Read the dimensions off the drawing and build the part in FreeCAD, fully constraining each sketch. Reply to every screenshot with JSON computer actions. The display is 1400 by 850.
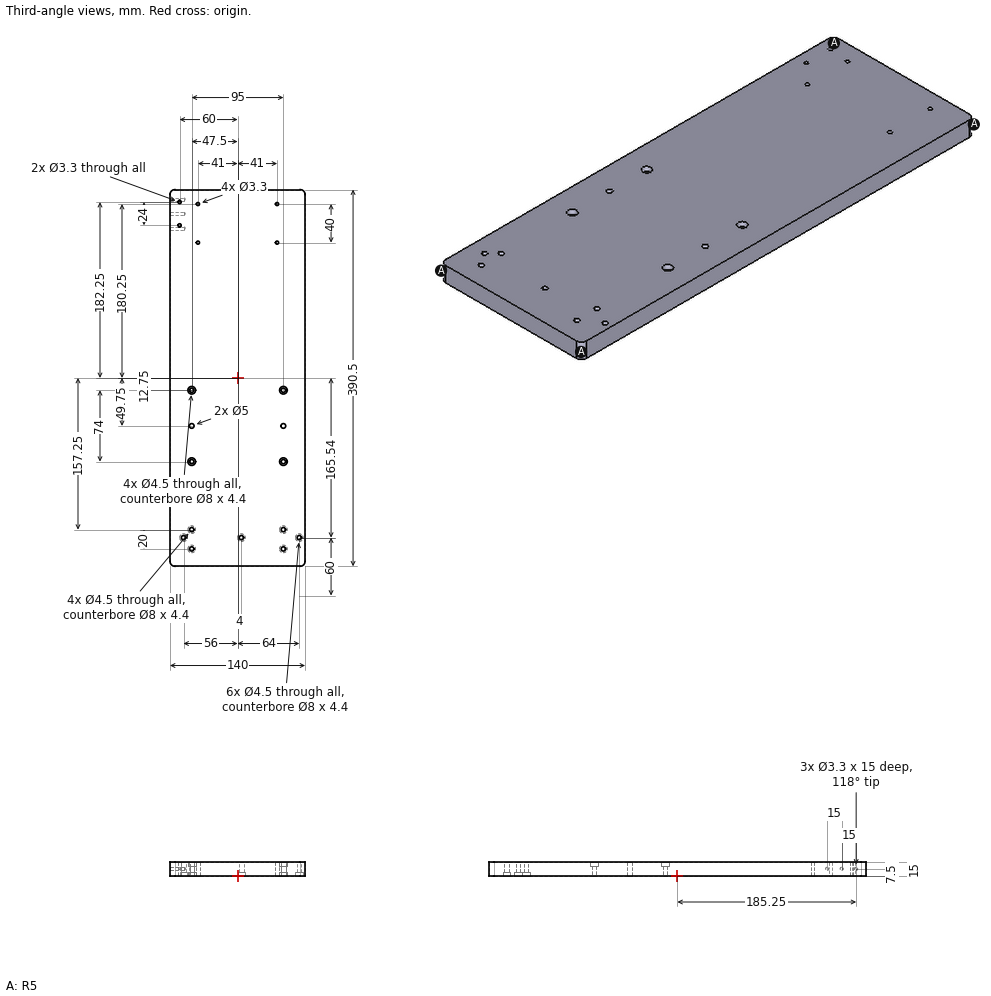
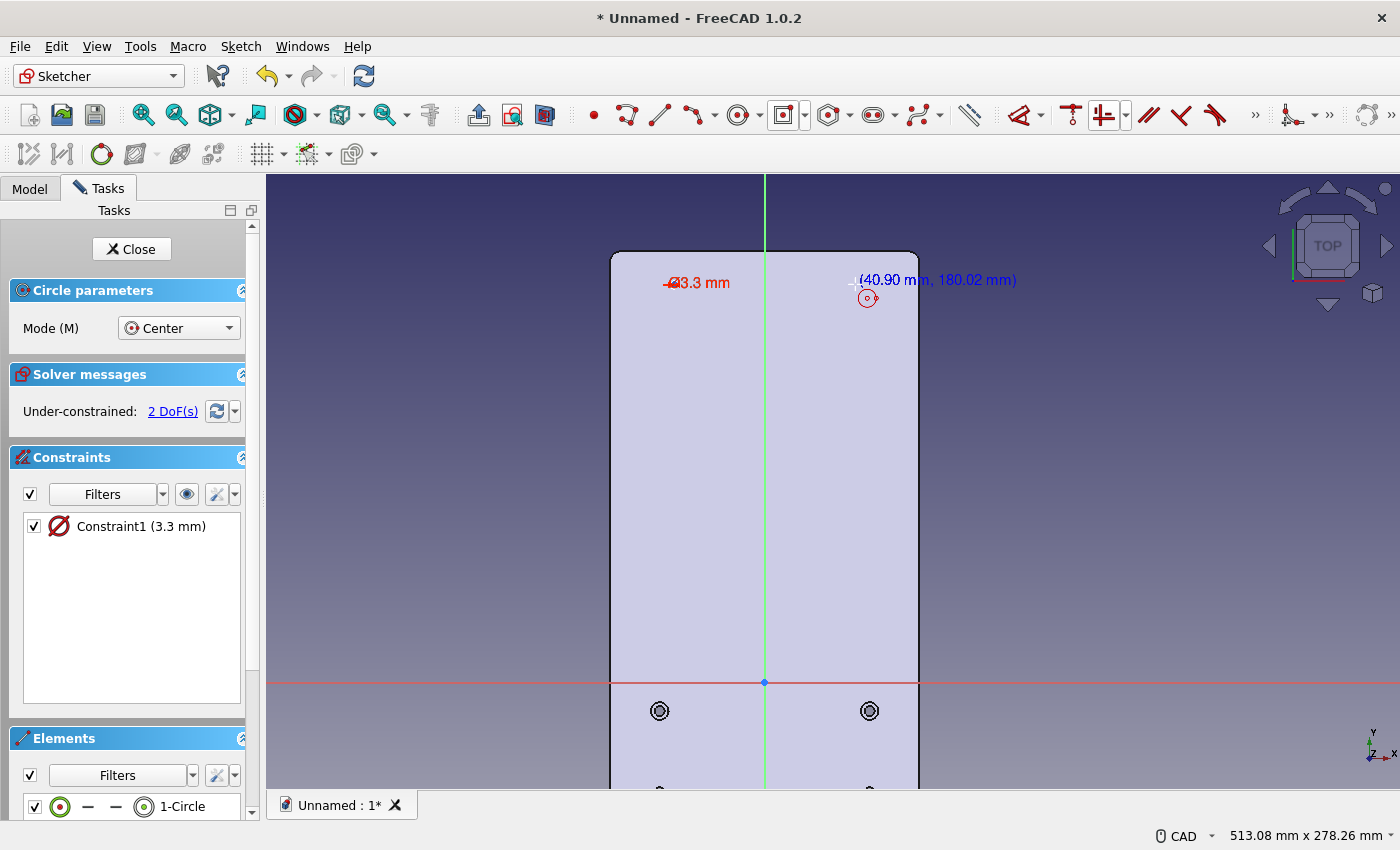
{"action": "left_click", "coordinate": [855, 284]}
{"action": "mouse_move", "coordinate": [858, 282]}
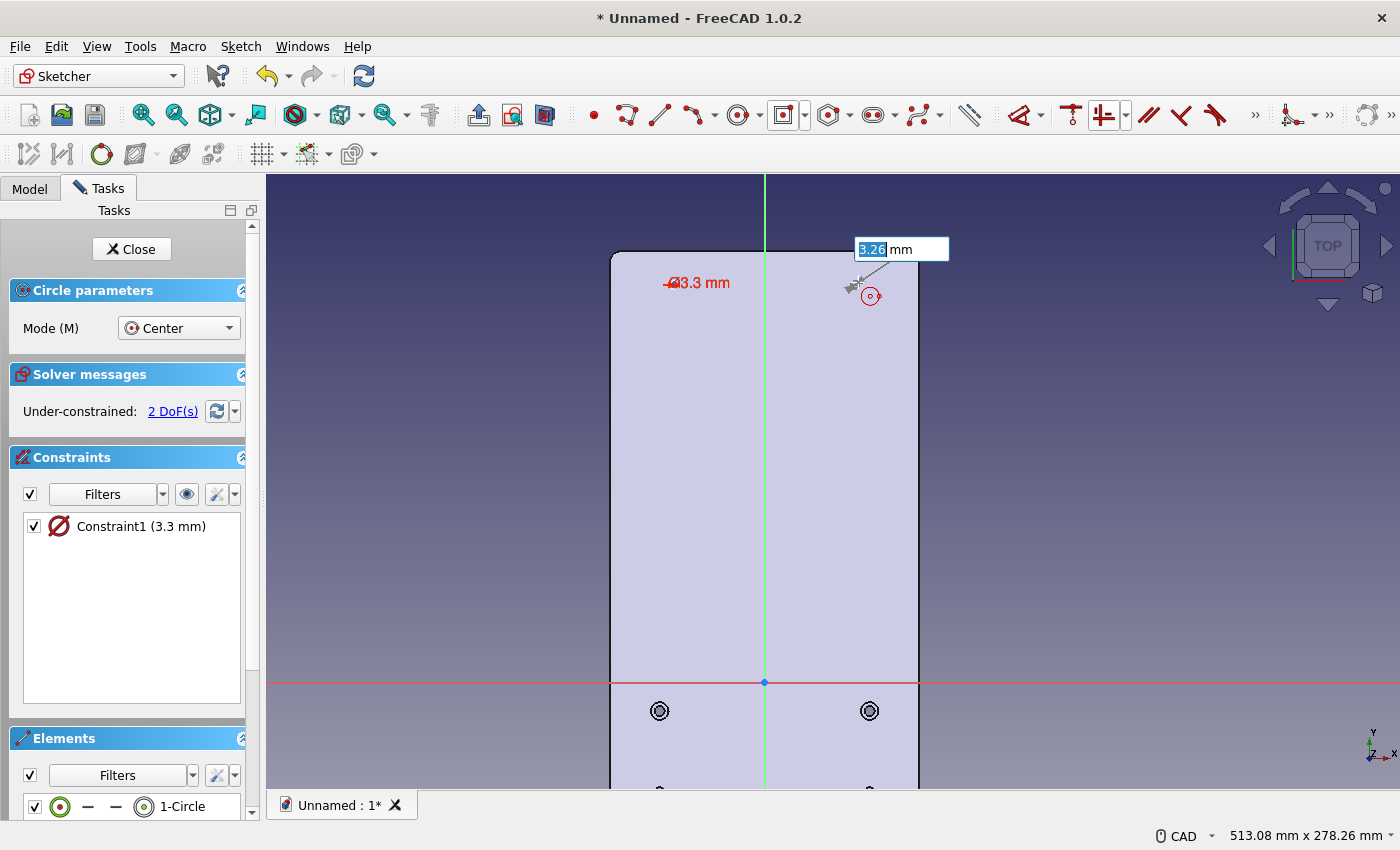
{"action": "type", "text": "3.3"}
{"action": "key", "text": "Return"}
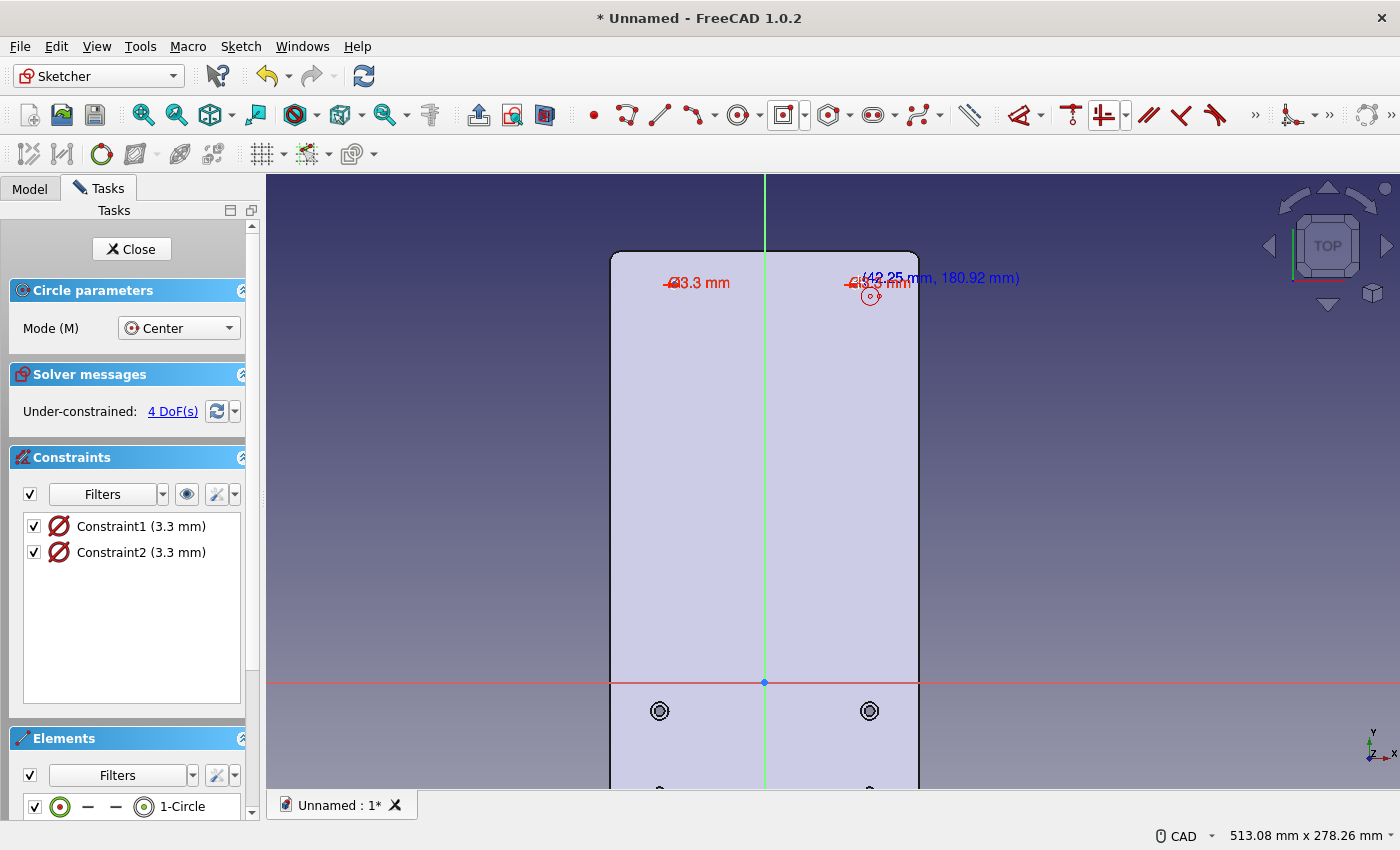
{"action": "scroll", "coordinate": [855, 373], "scroll_direction": "up", "scroll_amount": 10}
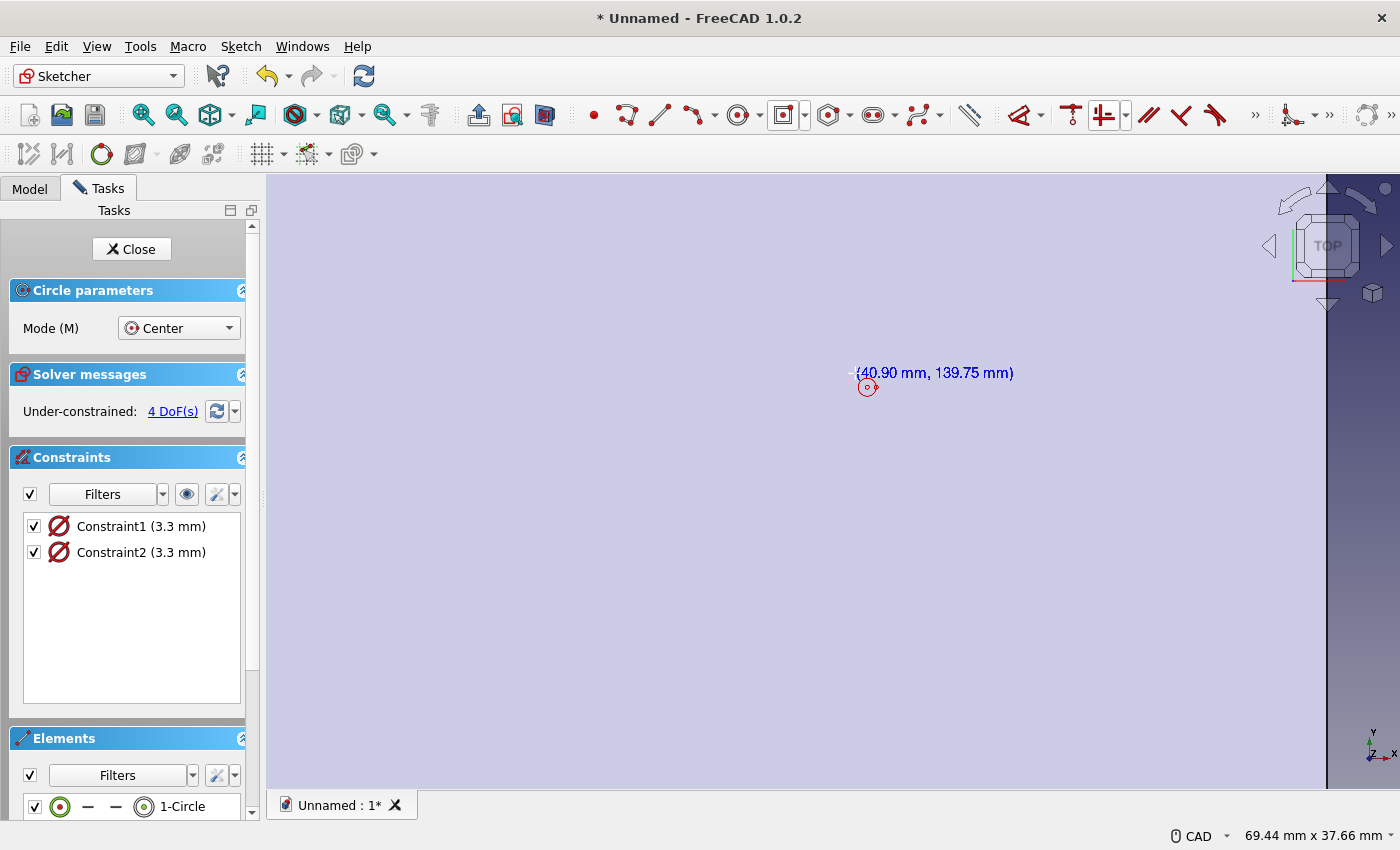
{"action": "scroll", "coordinate": [855, 373], "scroll_direction": "down", "scroll_amount": 10}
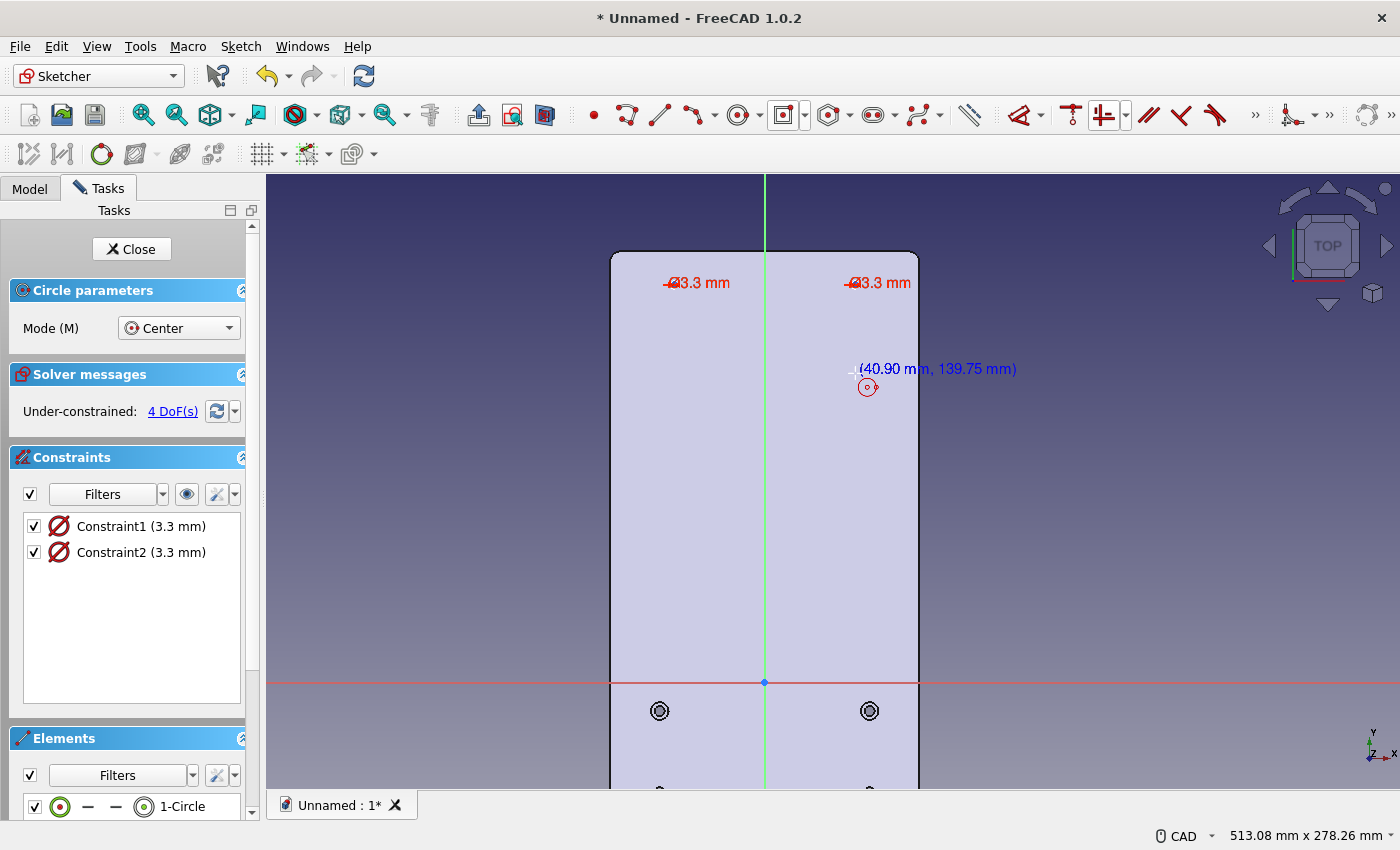
{"action": "left_click", "coordinate": [855, 373]}
{"action": "mouse_move", "coordinate": [858, 370]}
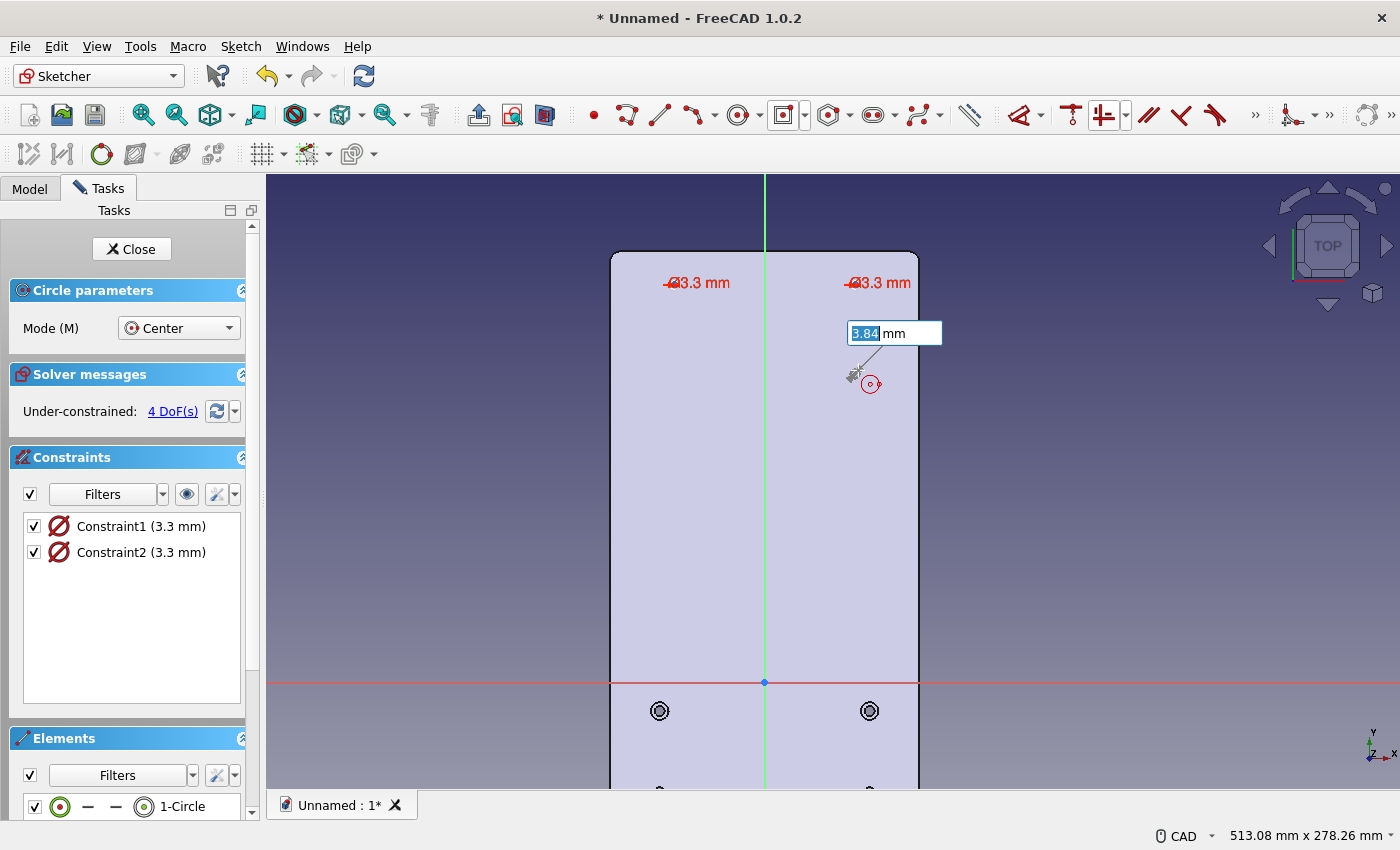
{"action": "type", "text": "3.3"}
{"action": "key", "text": "Return"}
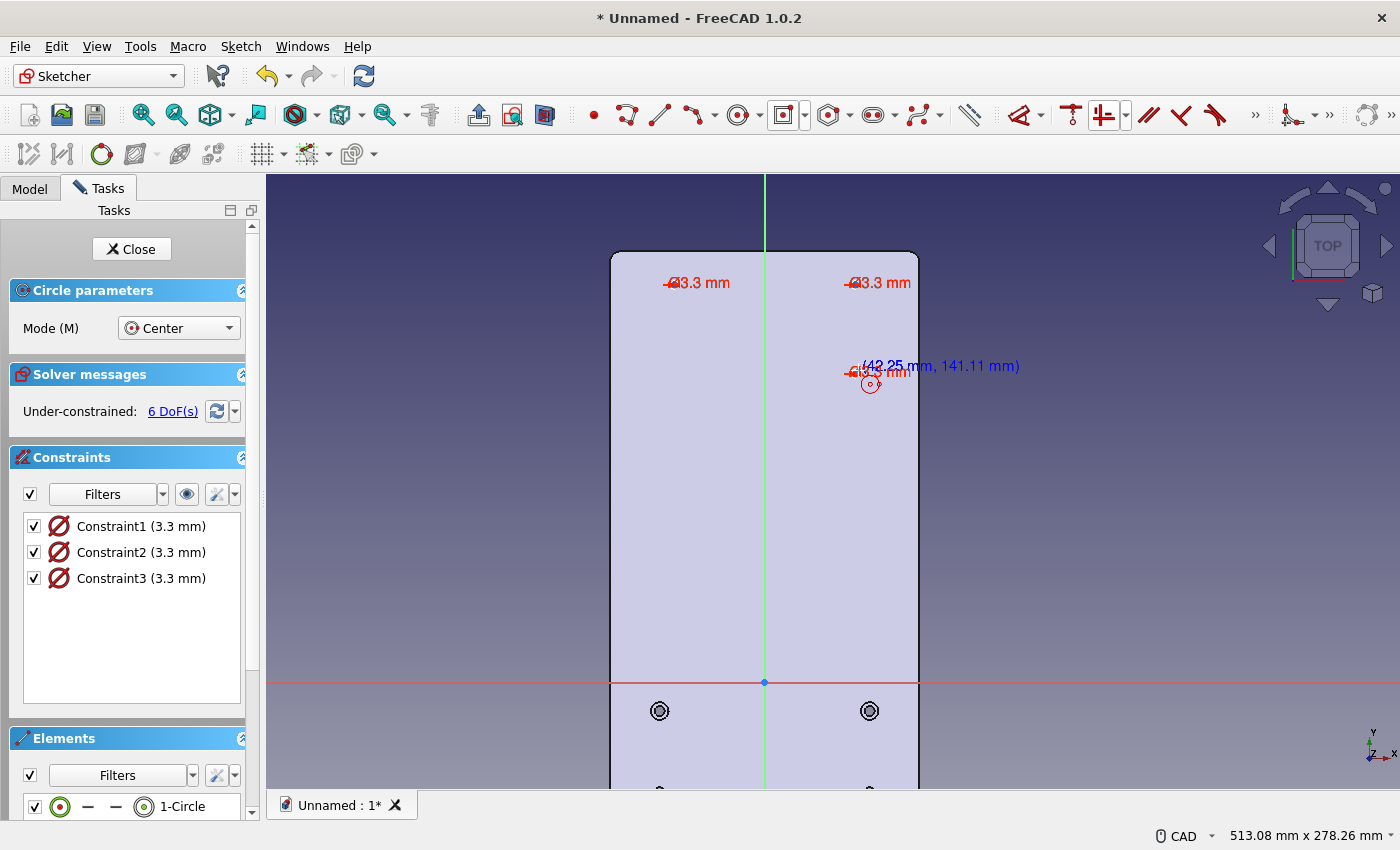
{"action": "scroll", "coordinate": [674, 373], "scroll_direction": "up", "scroll_amount": 10}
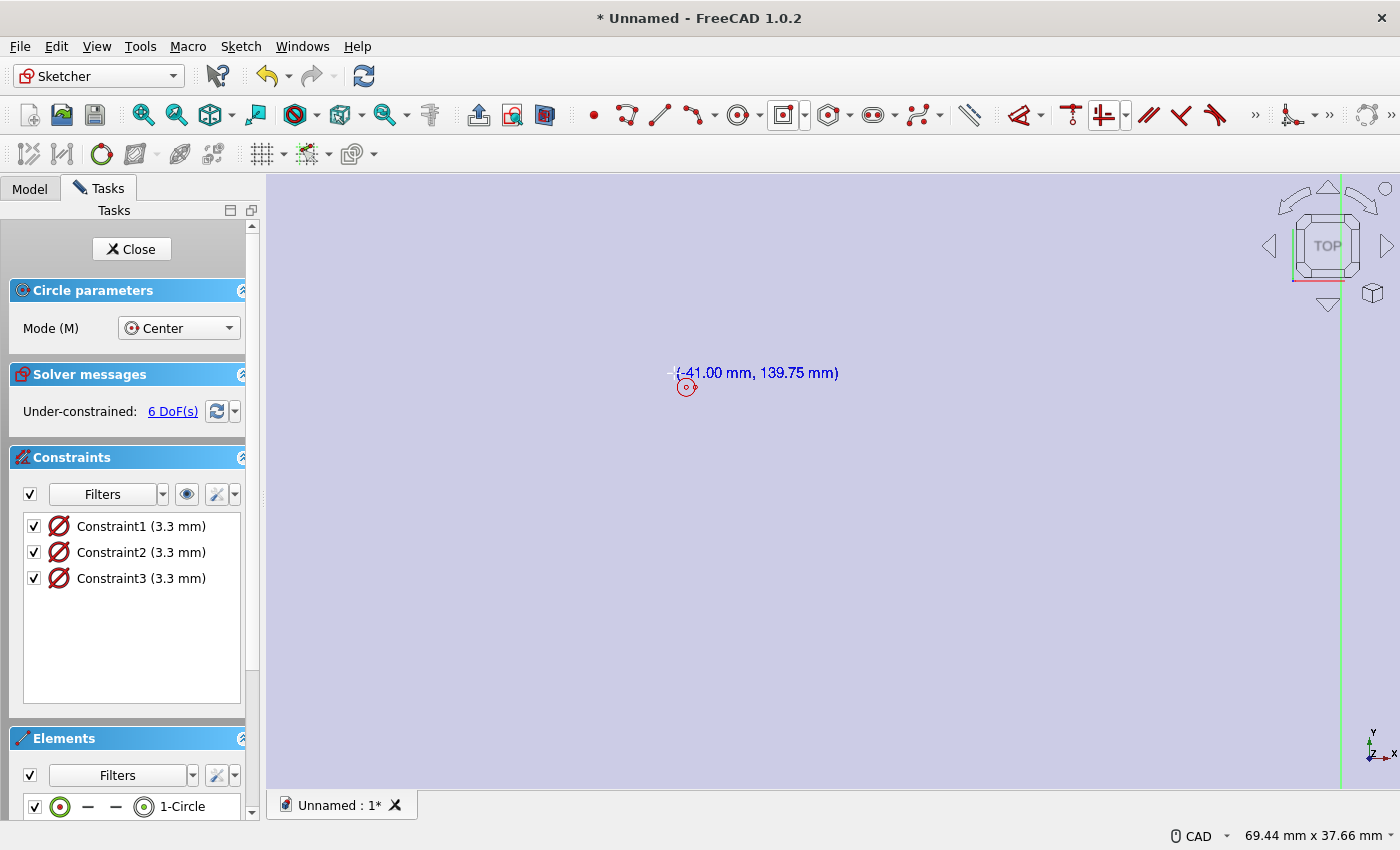
{"action": "scroll", "coordinate": [674, 373], "scroll_direction": "down", "scroll_amount": 10}